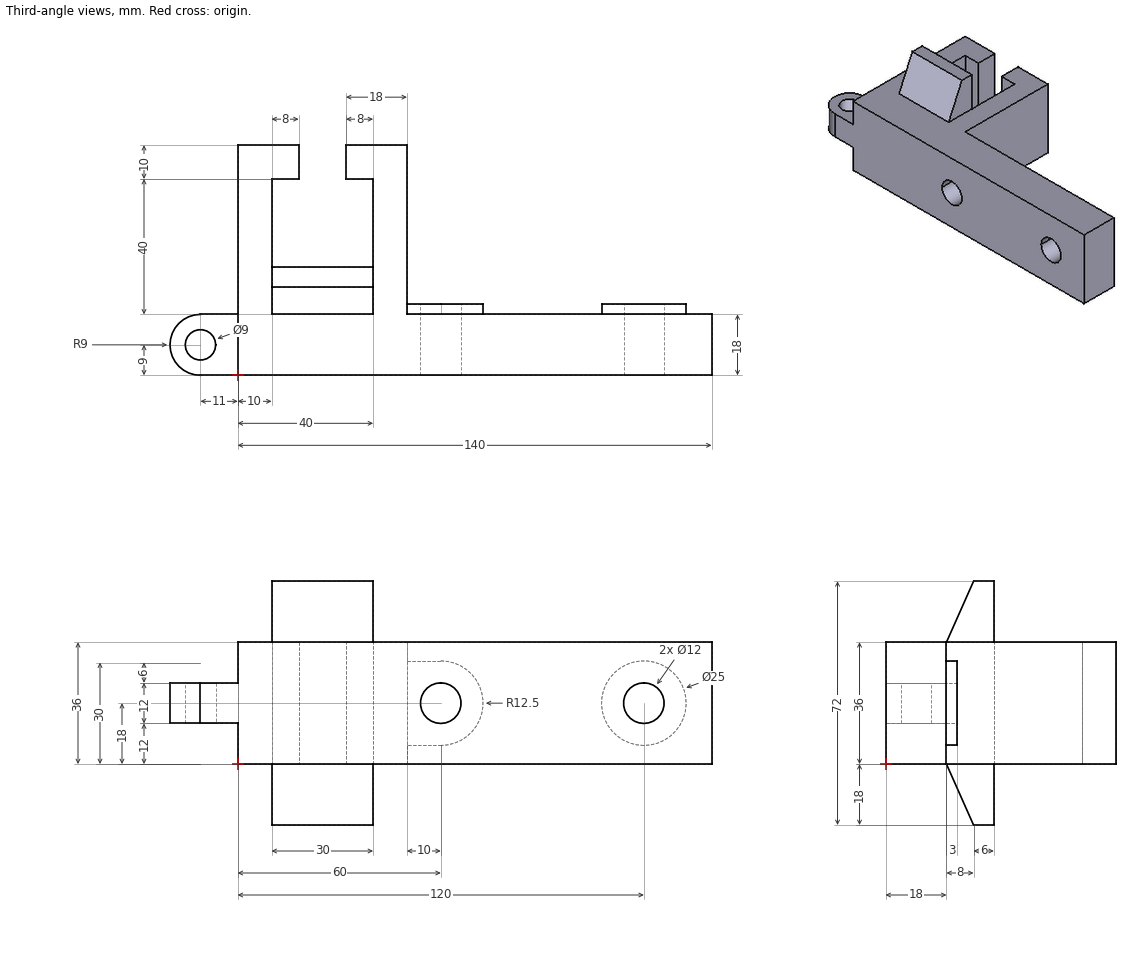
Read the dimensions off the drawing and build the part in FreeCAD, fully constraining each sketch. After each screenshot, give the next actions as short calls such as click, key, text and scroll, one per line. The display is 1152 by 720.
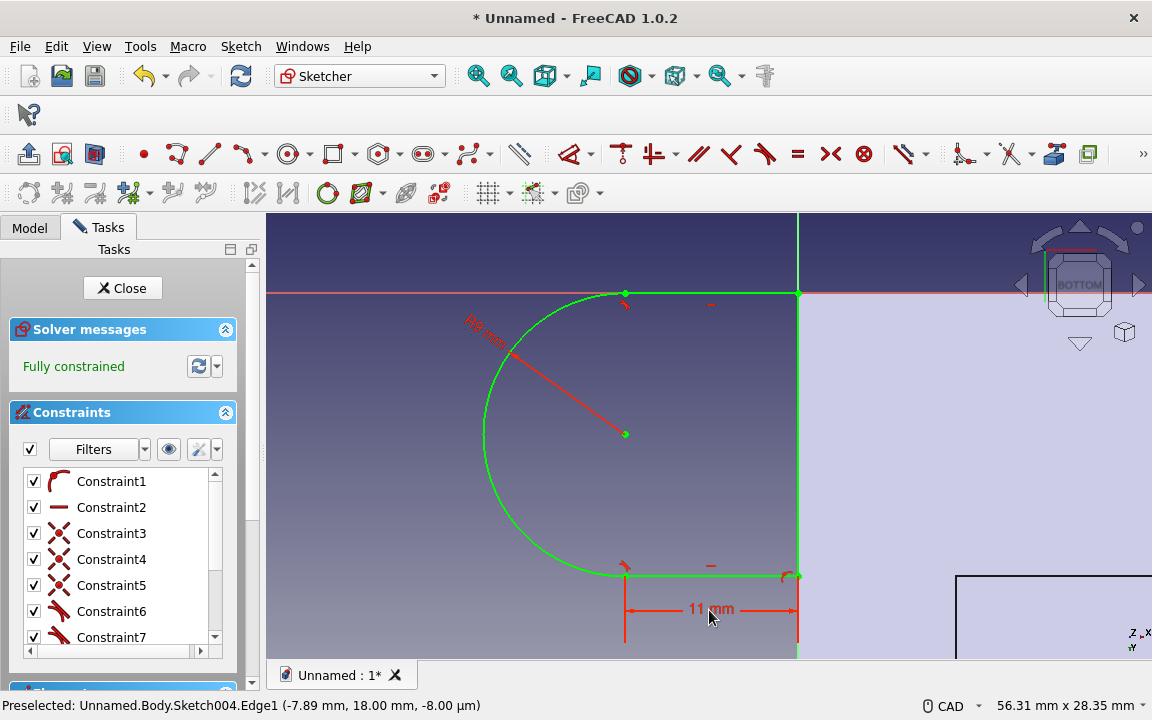
click(123, 288)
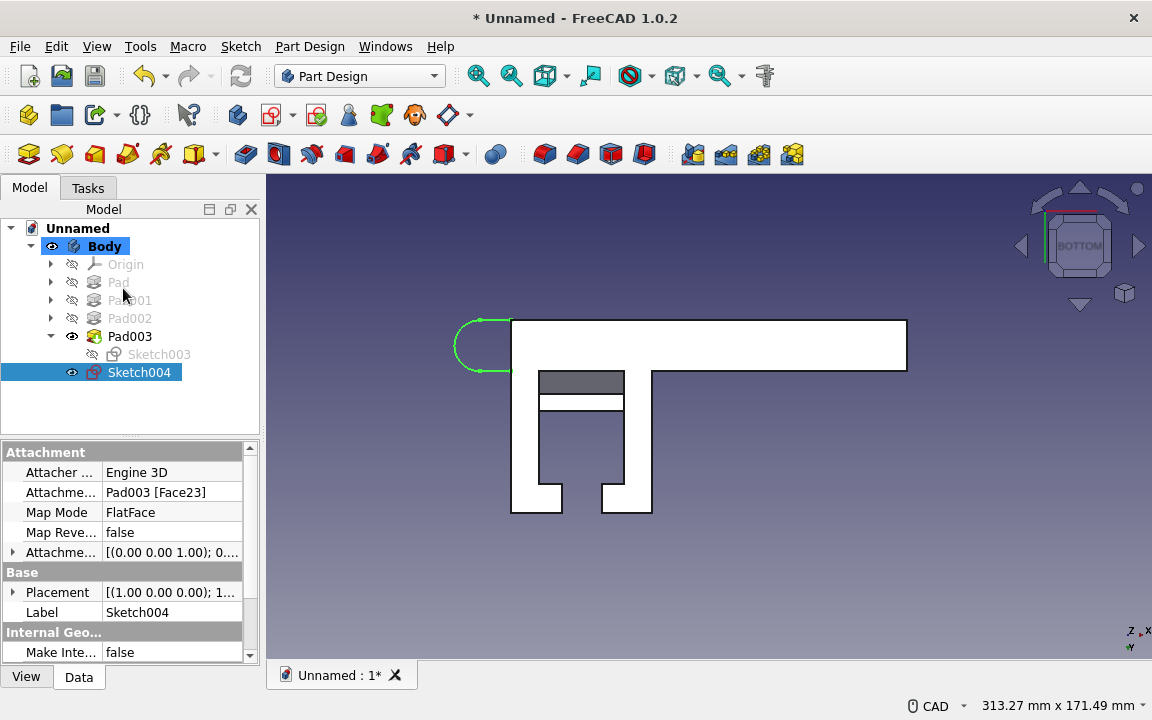
click(29, 154)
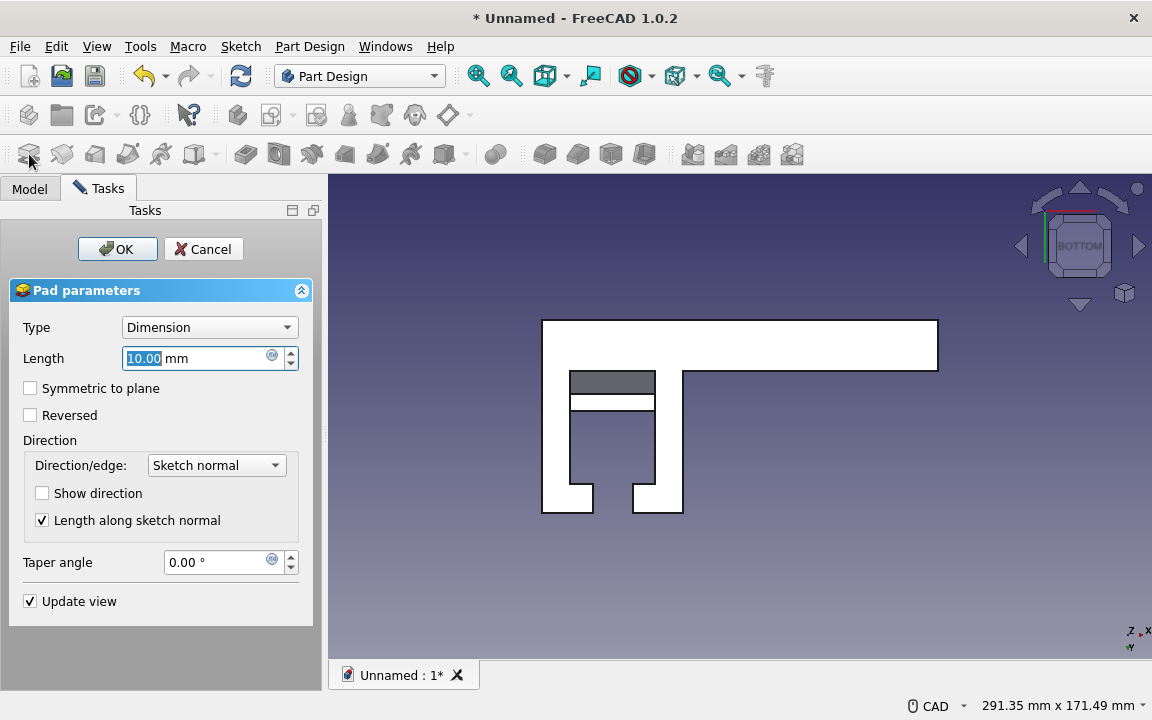
text(30)
key(Tab)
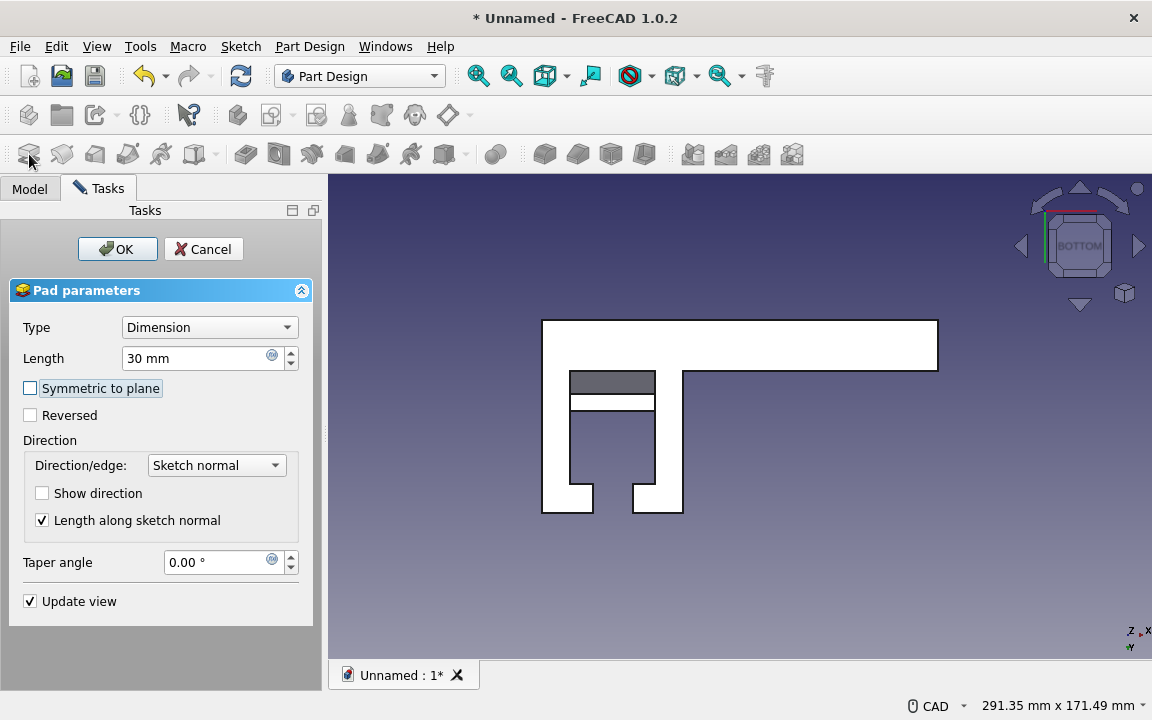
click(31, 415)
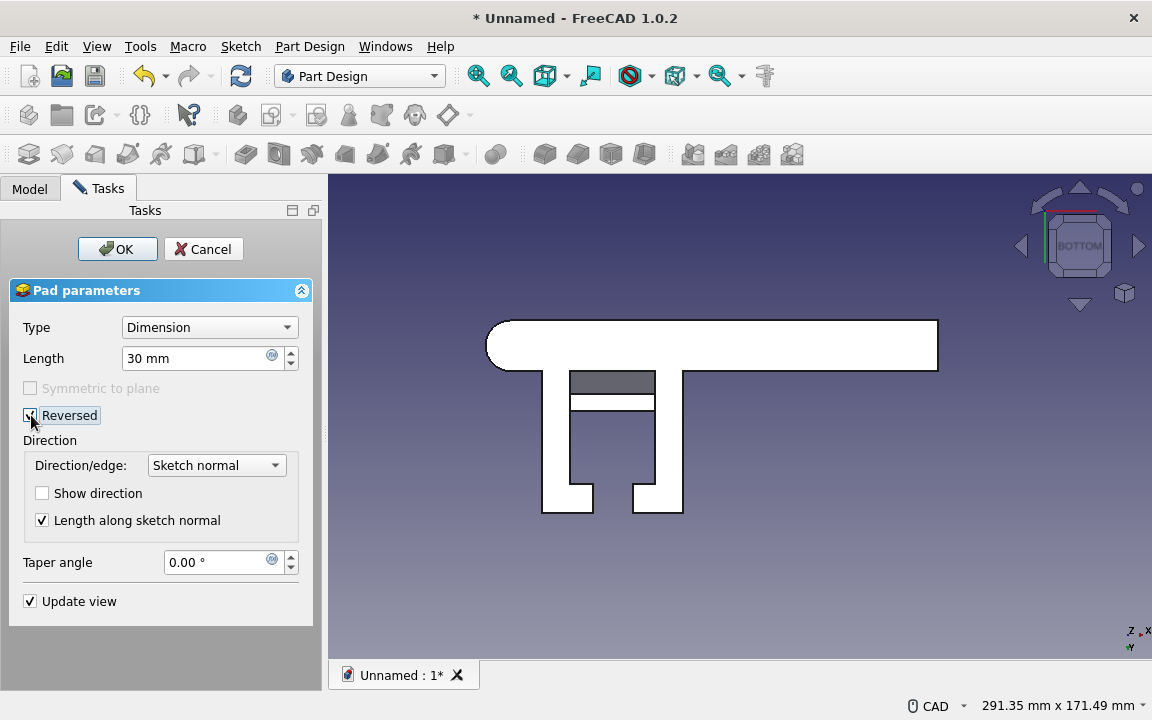
click(118, 249)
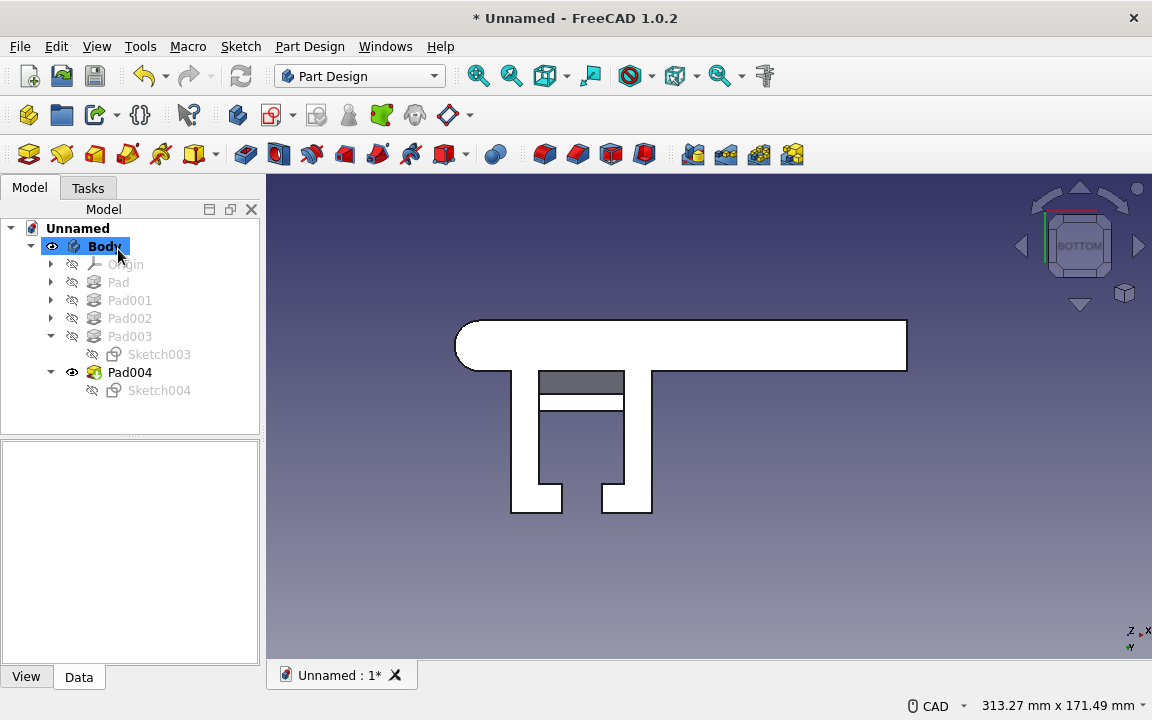
click(270, 116)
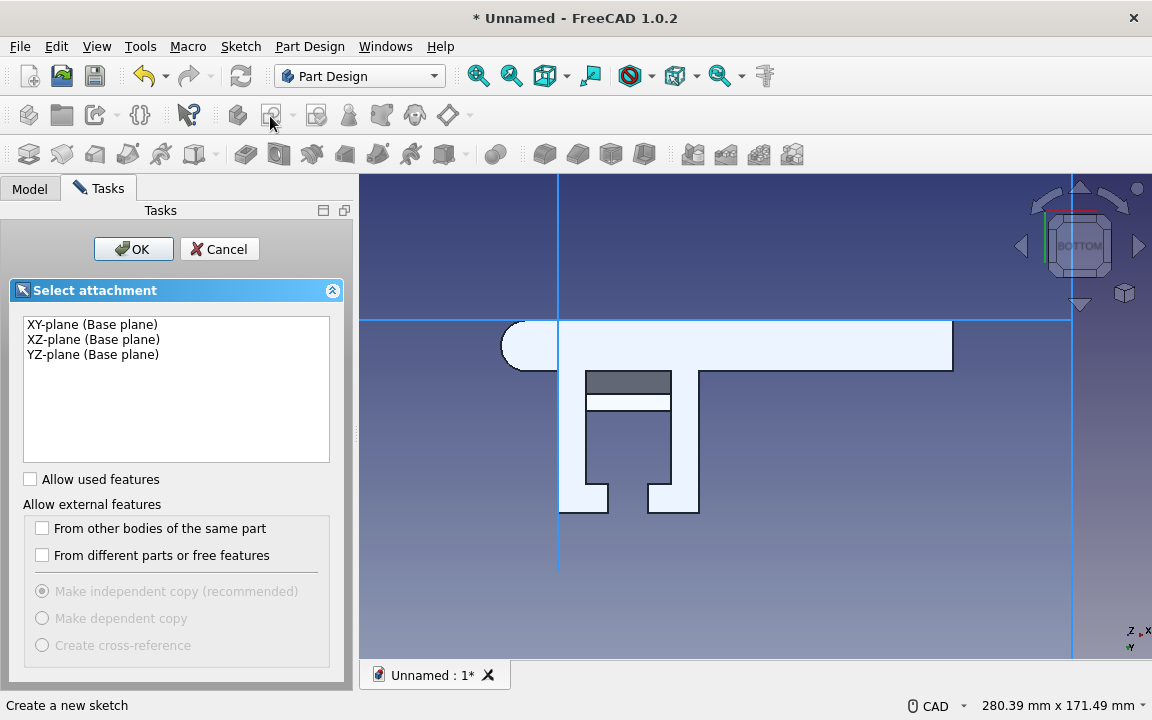
click(84, 324)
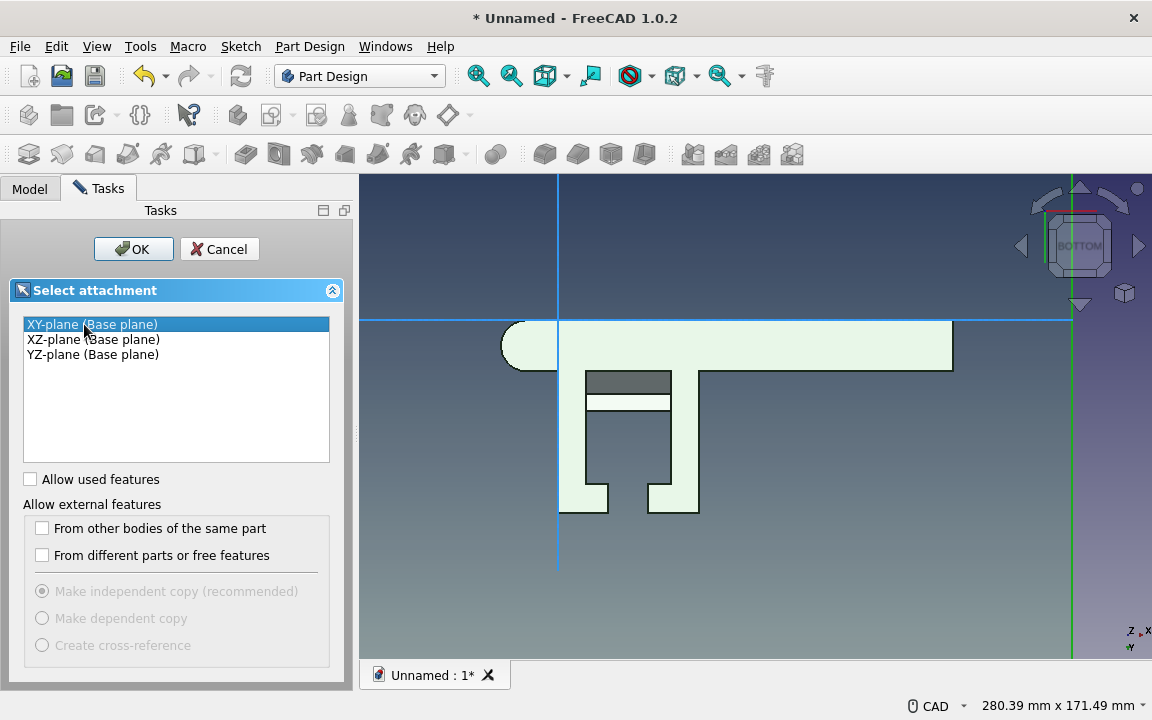
click(134, 249)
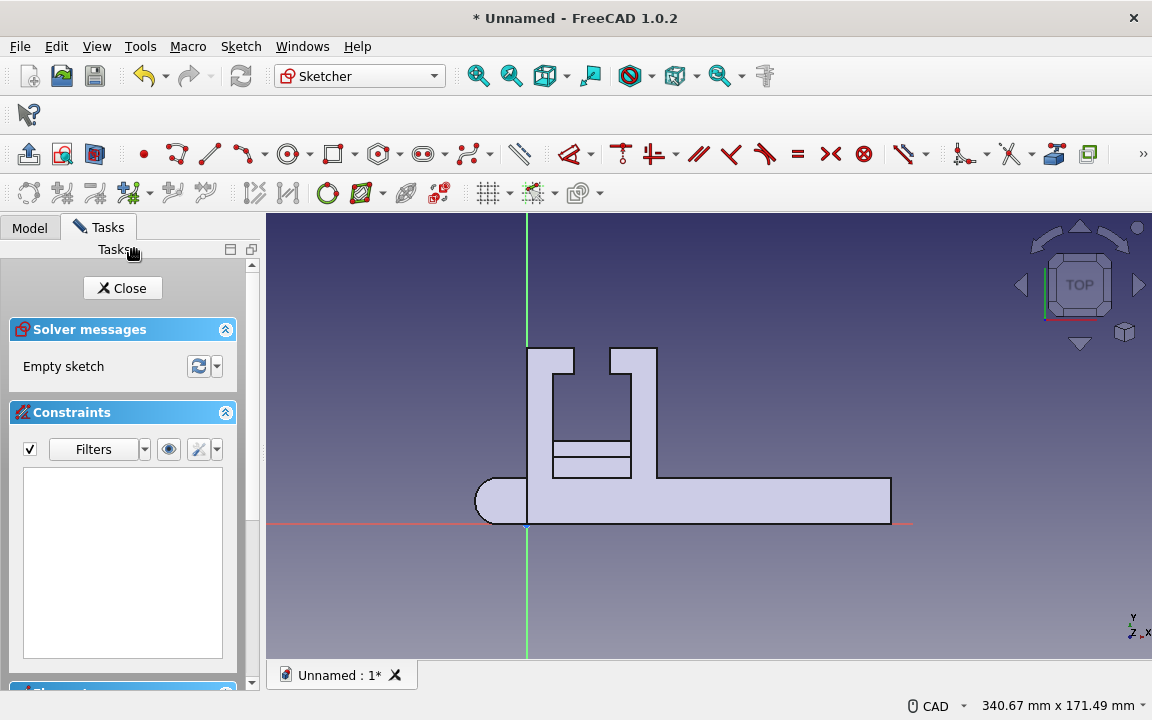
click(95, 154)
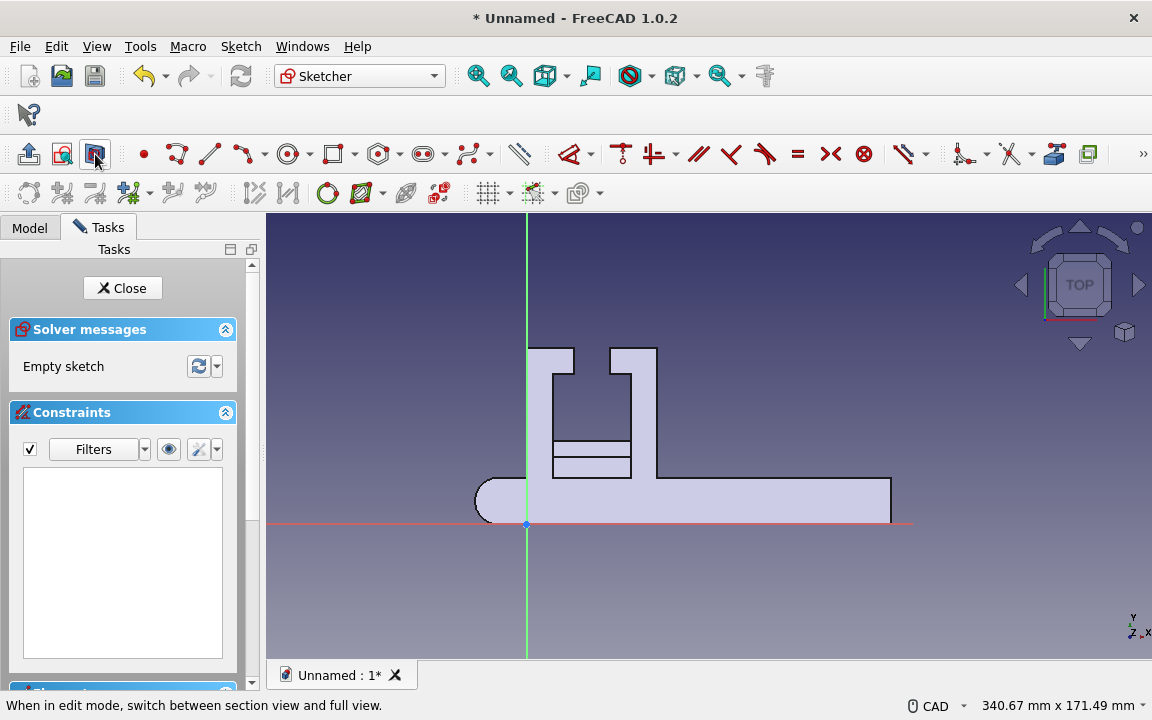
scroll(473, 514, up, 9)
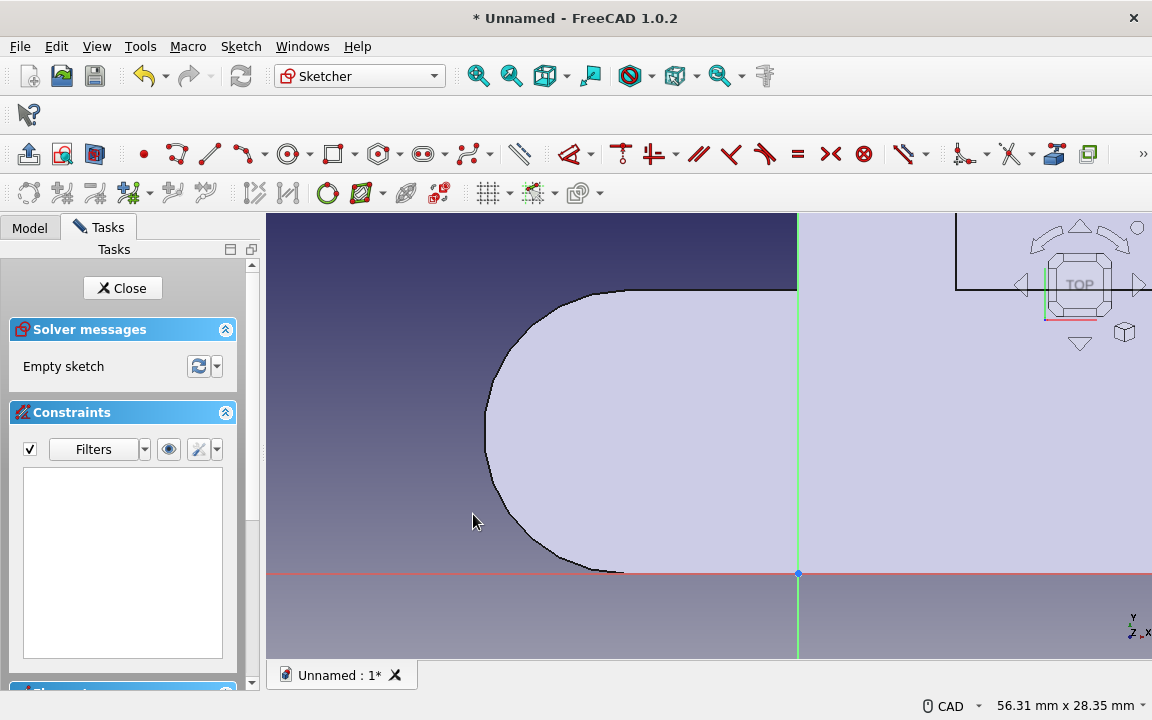
key(g)
key(m)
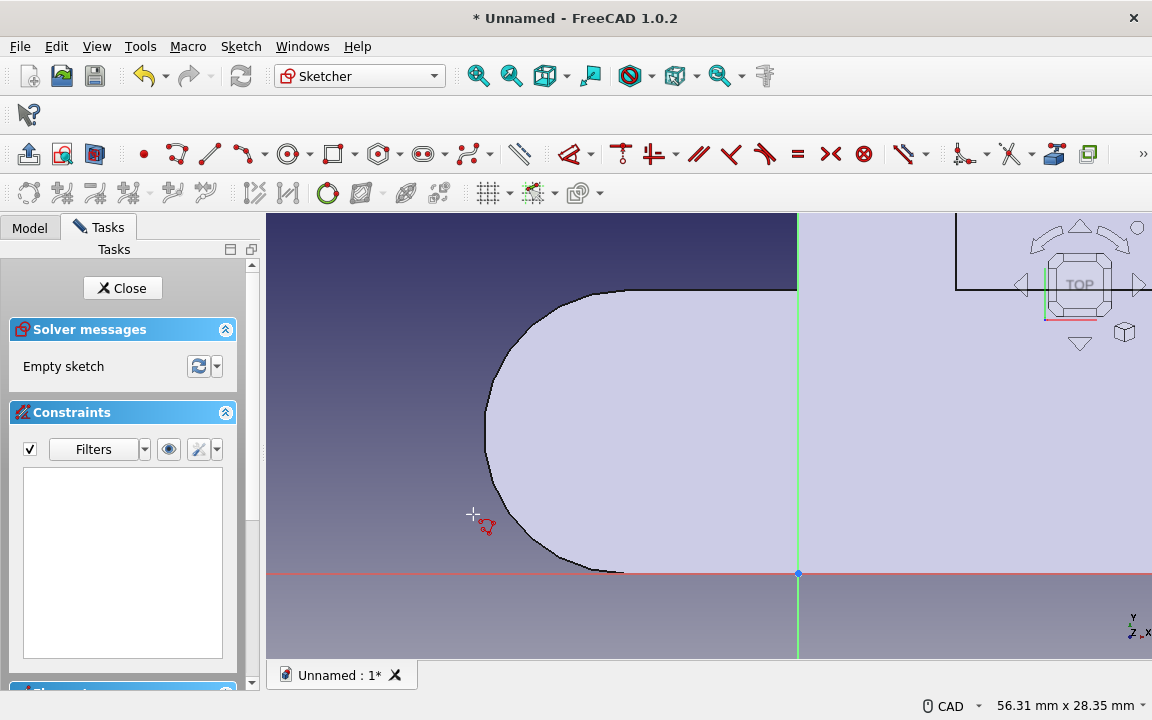
click(625, 290)
click(798, 290)
click(798, 574)
click(625, 565)
right_click(625, 565)